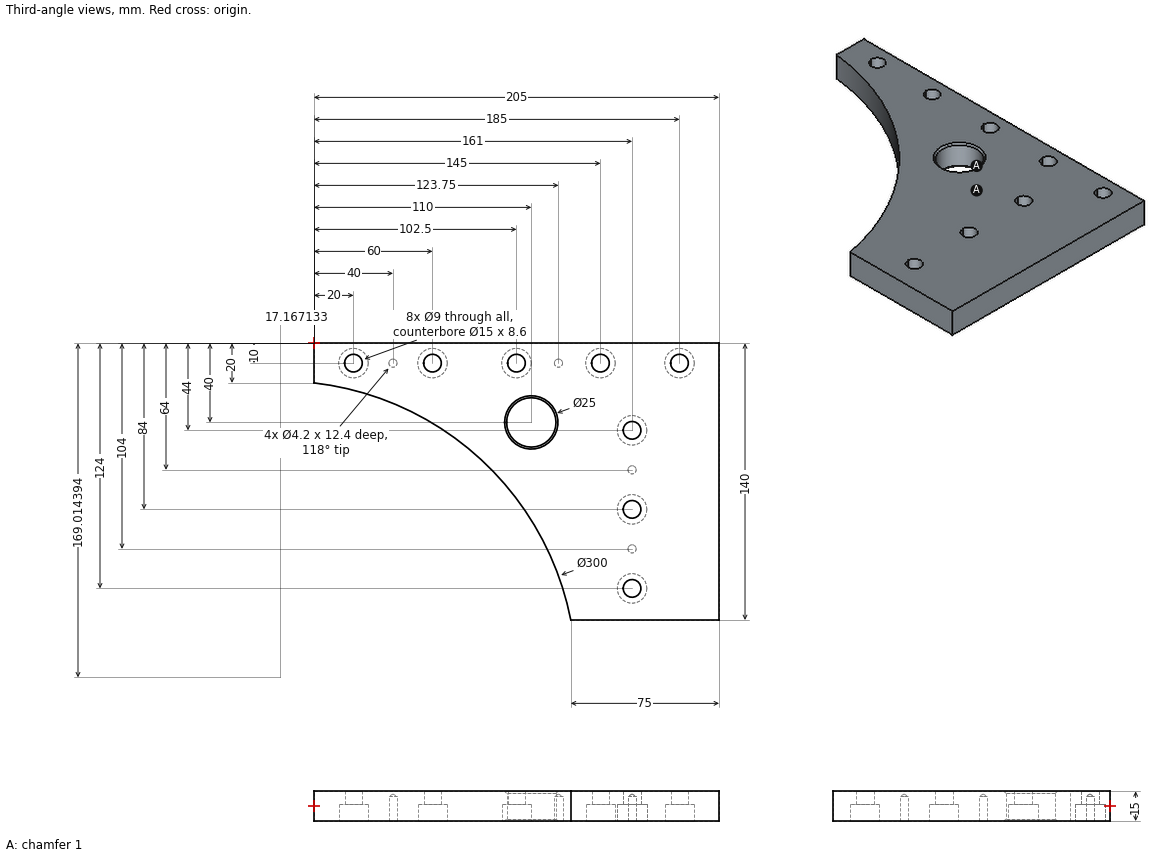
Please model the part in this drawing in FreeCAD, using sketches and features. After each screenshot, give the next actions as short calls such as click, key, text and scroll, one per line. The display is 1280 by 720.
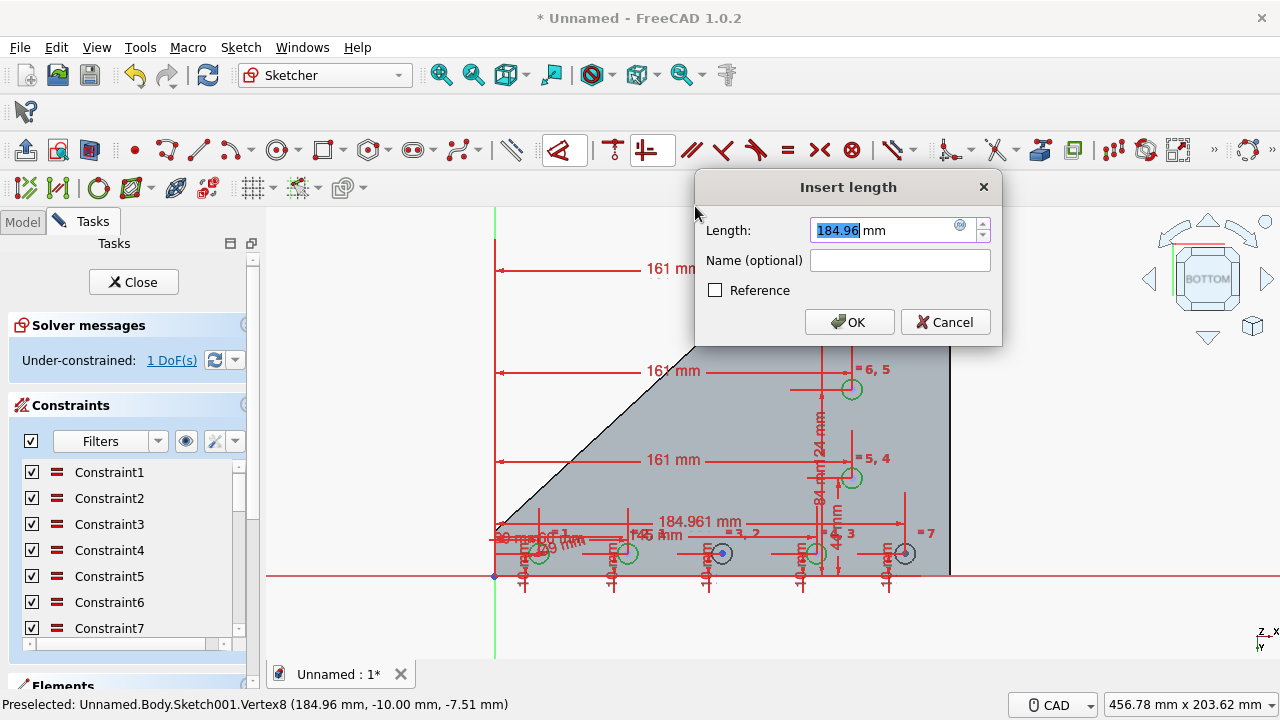
text(185)
key(Return)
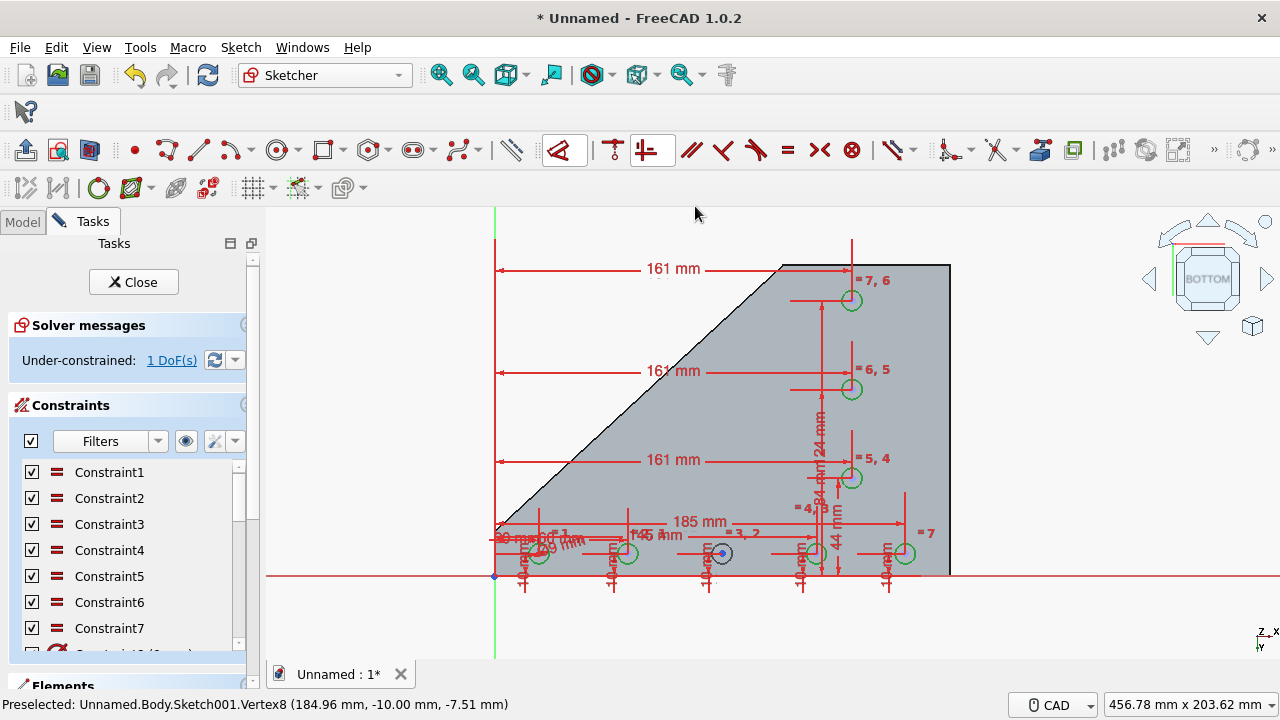
click(722, 554)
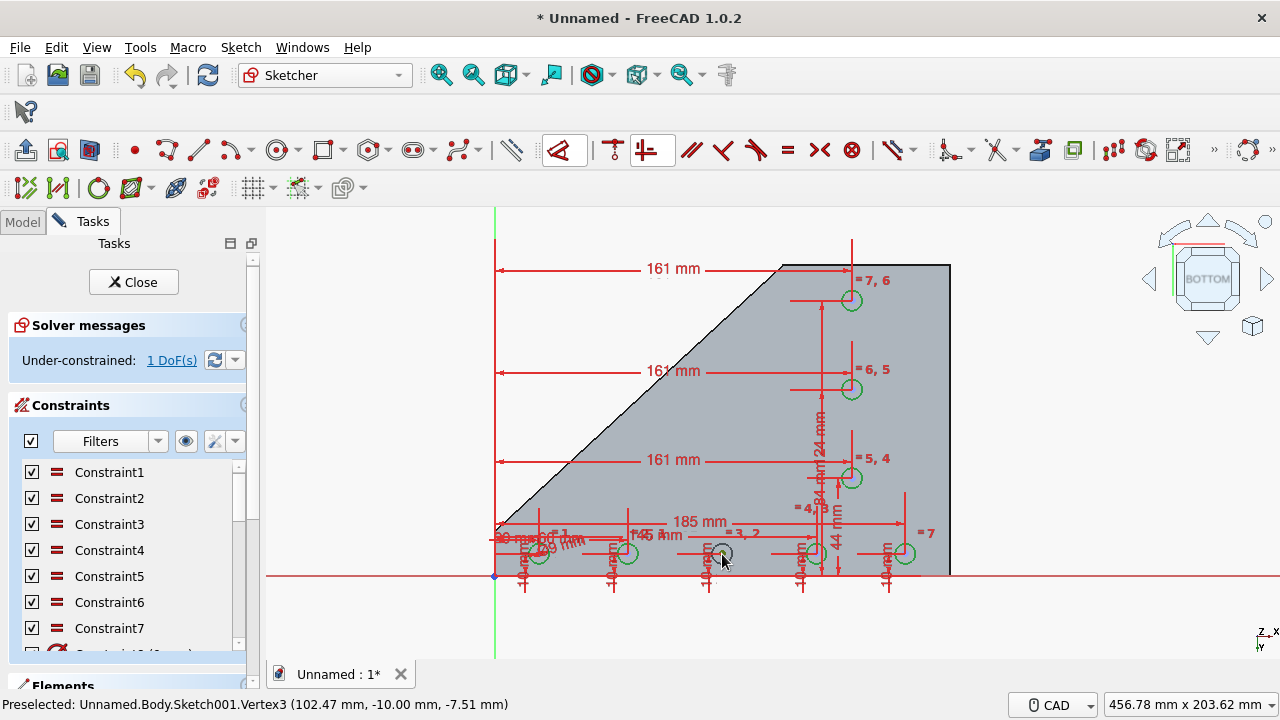
click(582, 150)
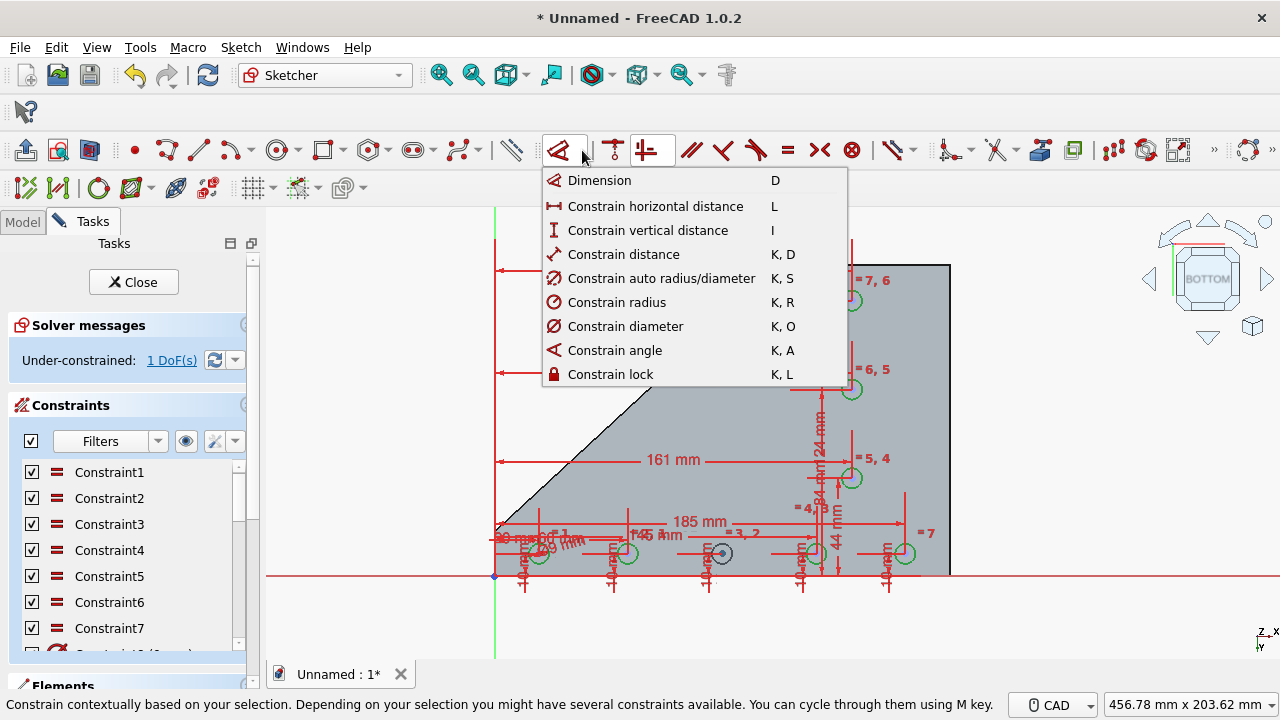
click(695, 206)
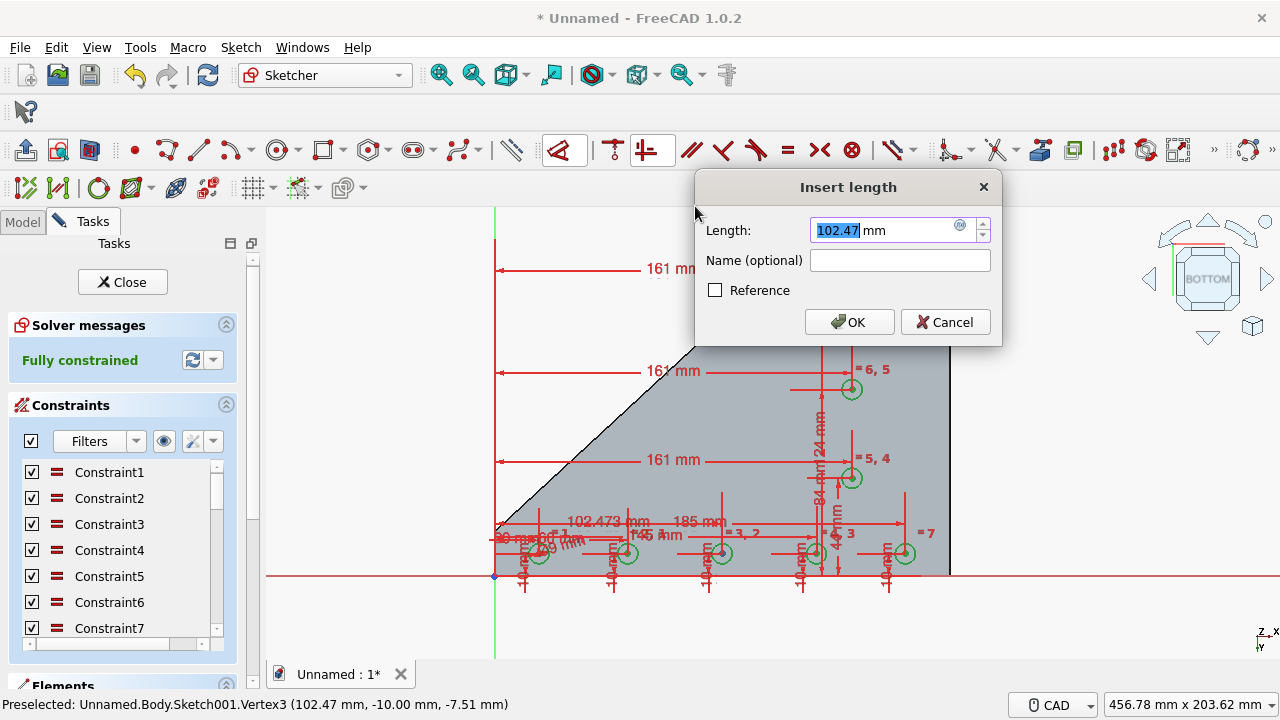
text(102.5)
key(Return)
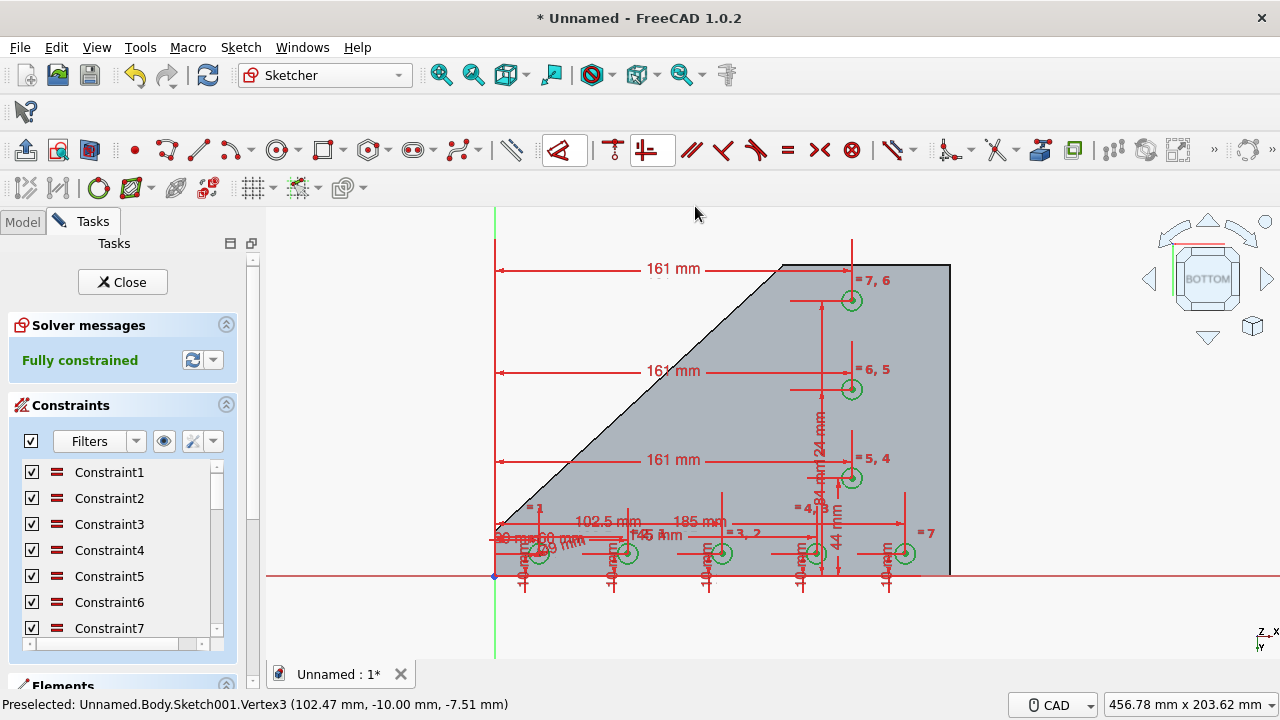
click(123, 282)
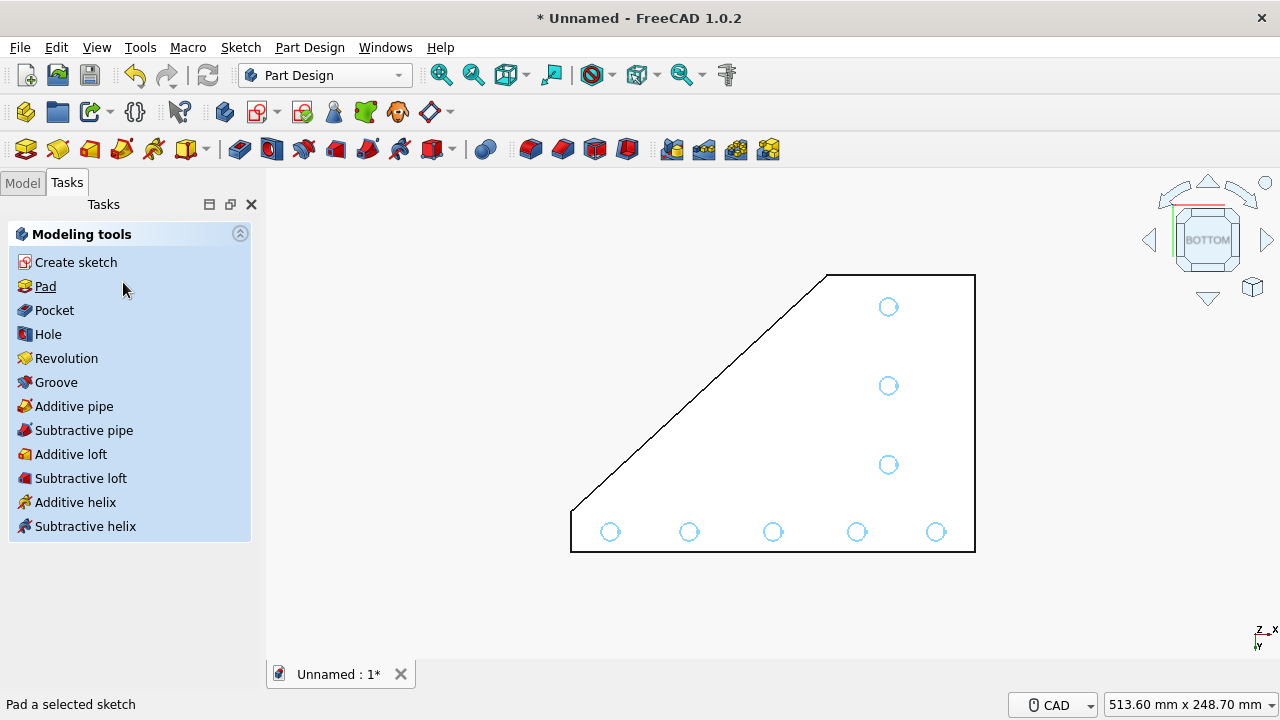
click(272, 150)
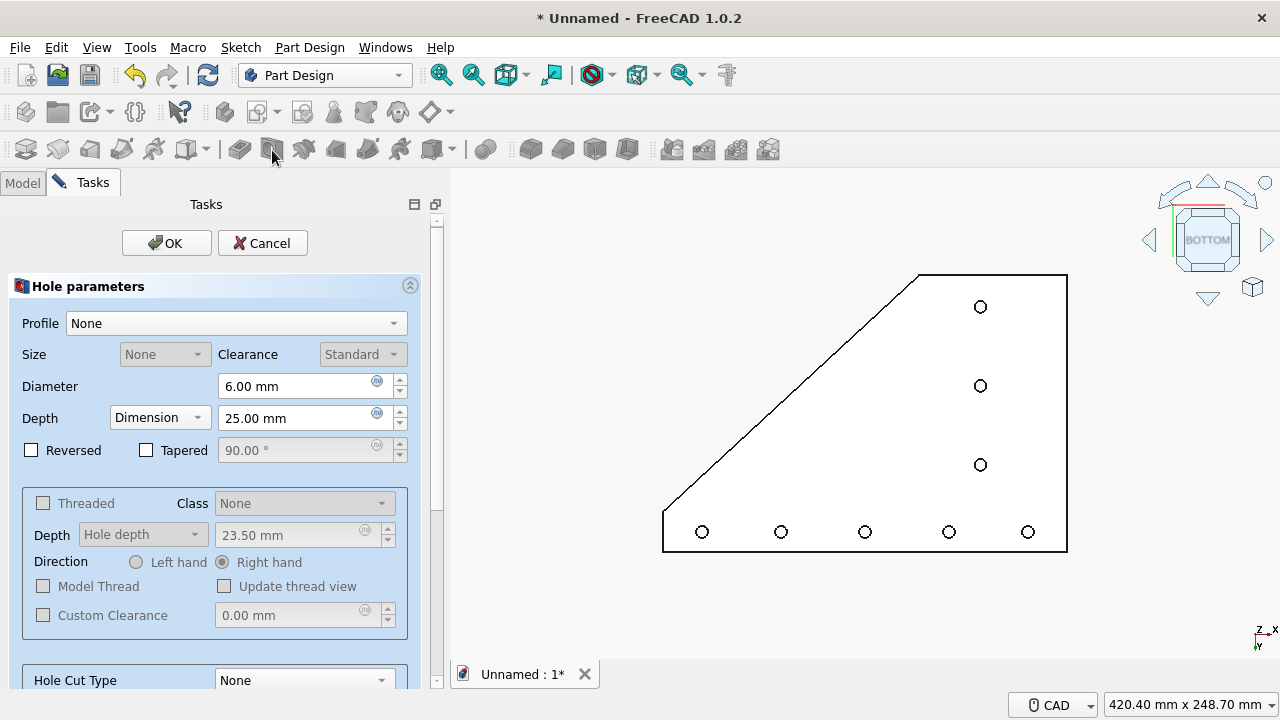
triple_click(305, 386)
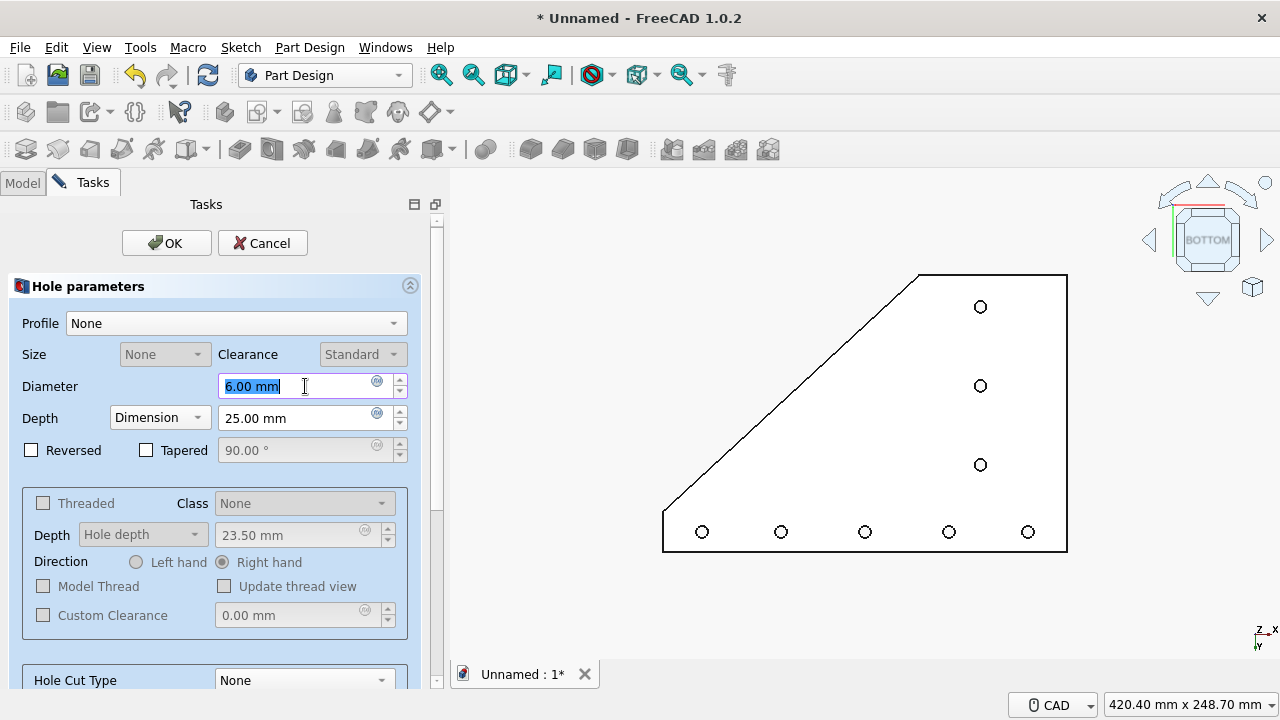
text(9)
key(Tab)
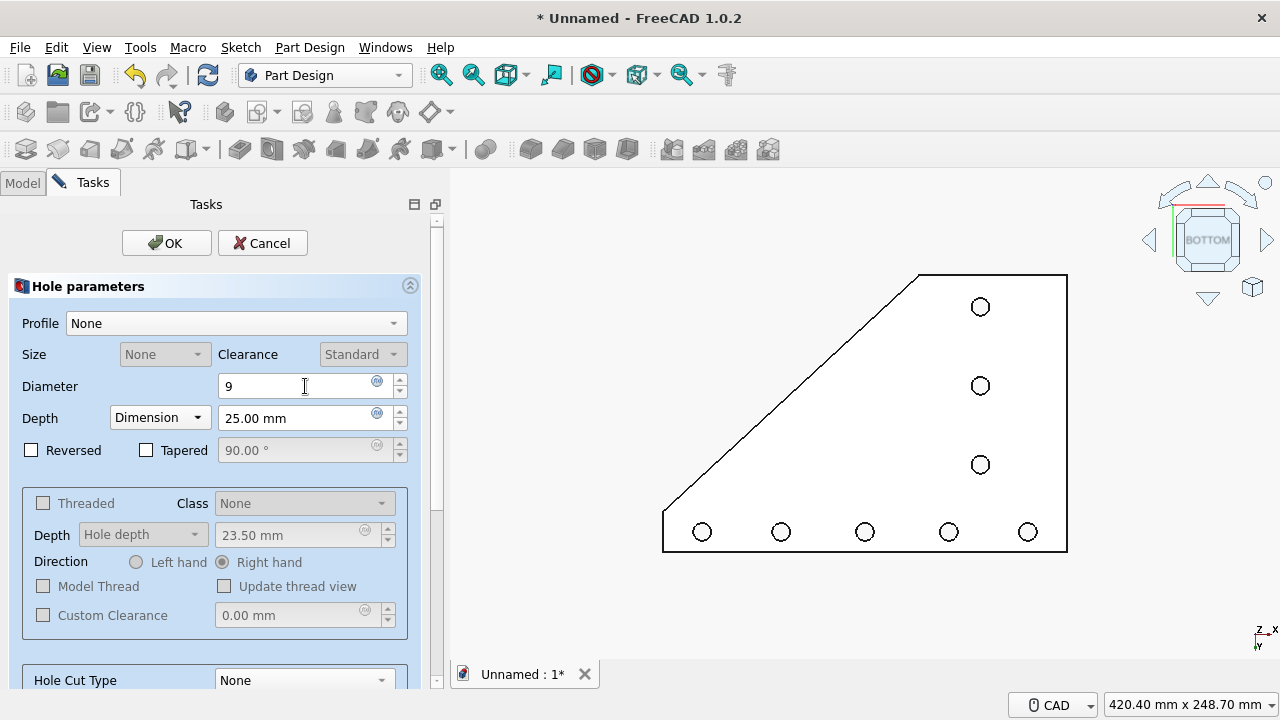
click(161, 418)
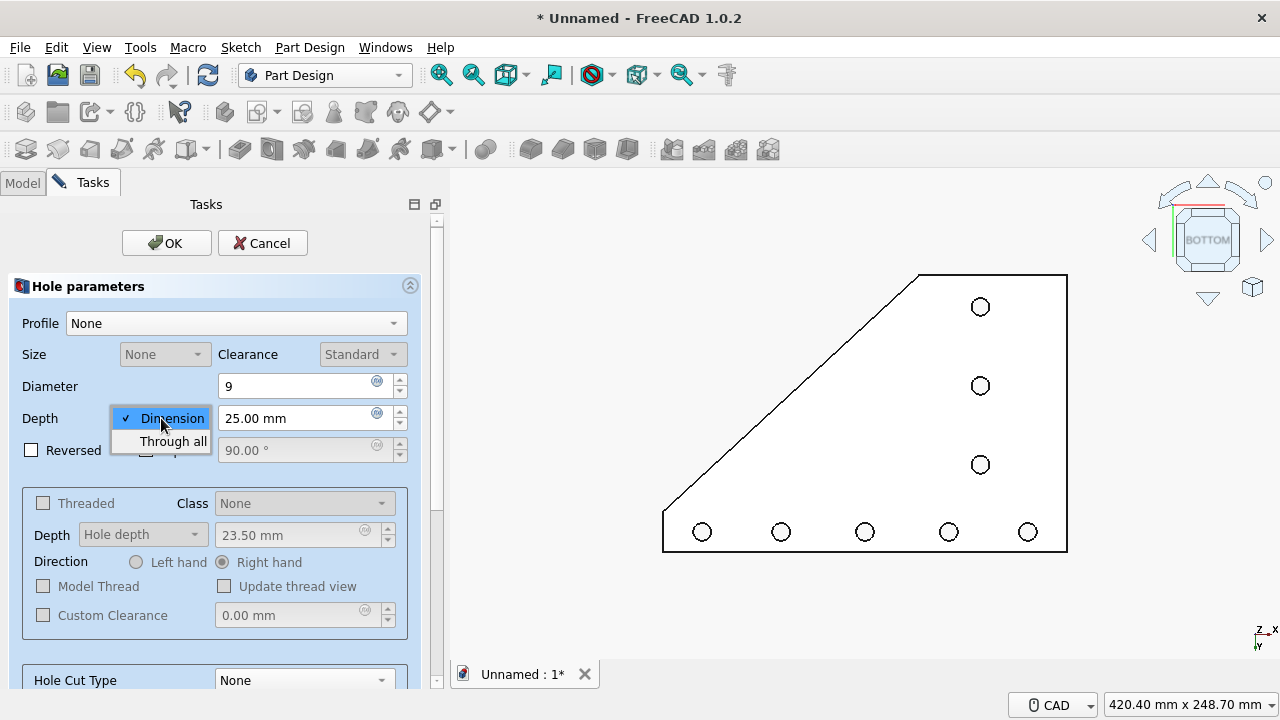
click(160, 442)